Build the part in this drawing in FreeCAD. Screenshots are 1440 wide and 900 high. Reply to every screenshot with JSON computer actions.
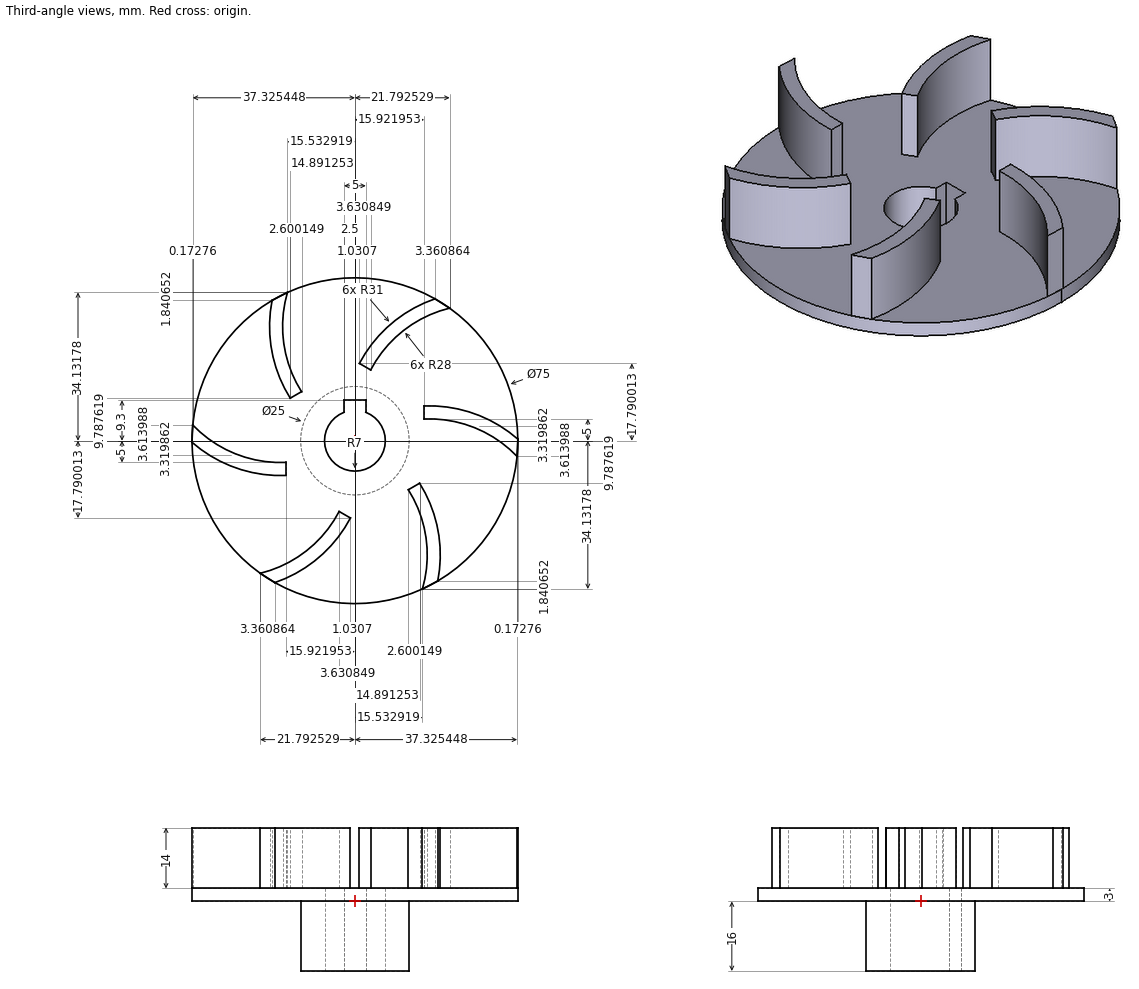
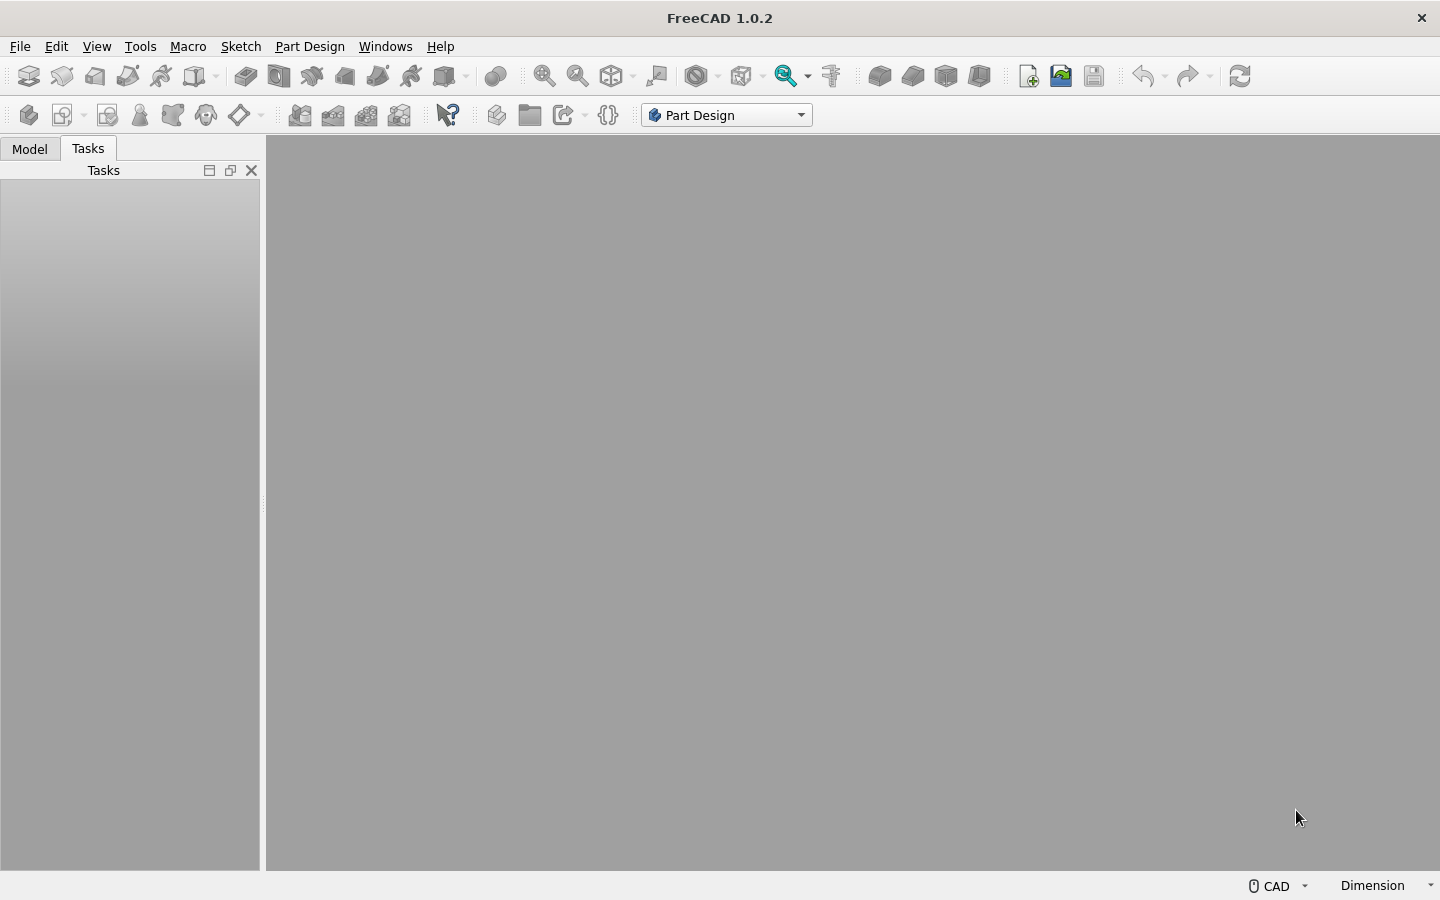
{"action": "key", "text": "ctrl+n"}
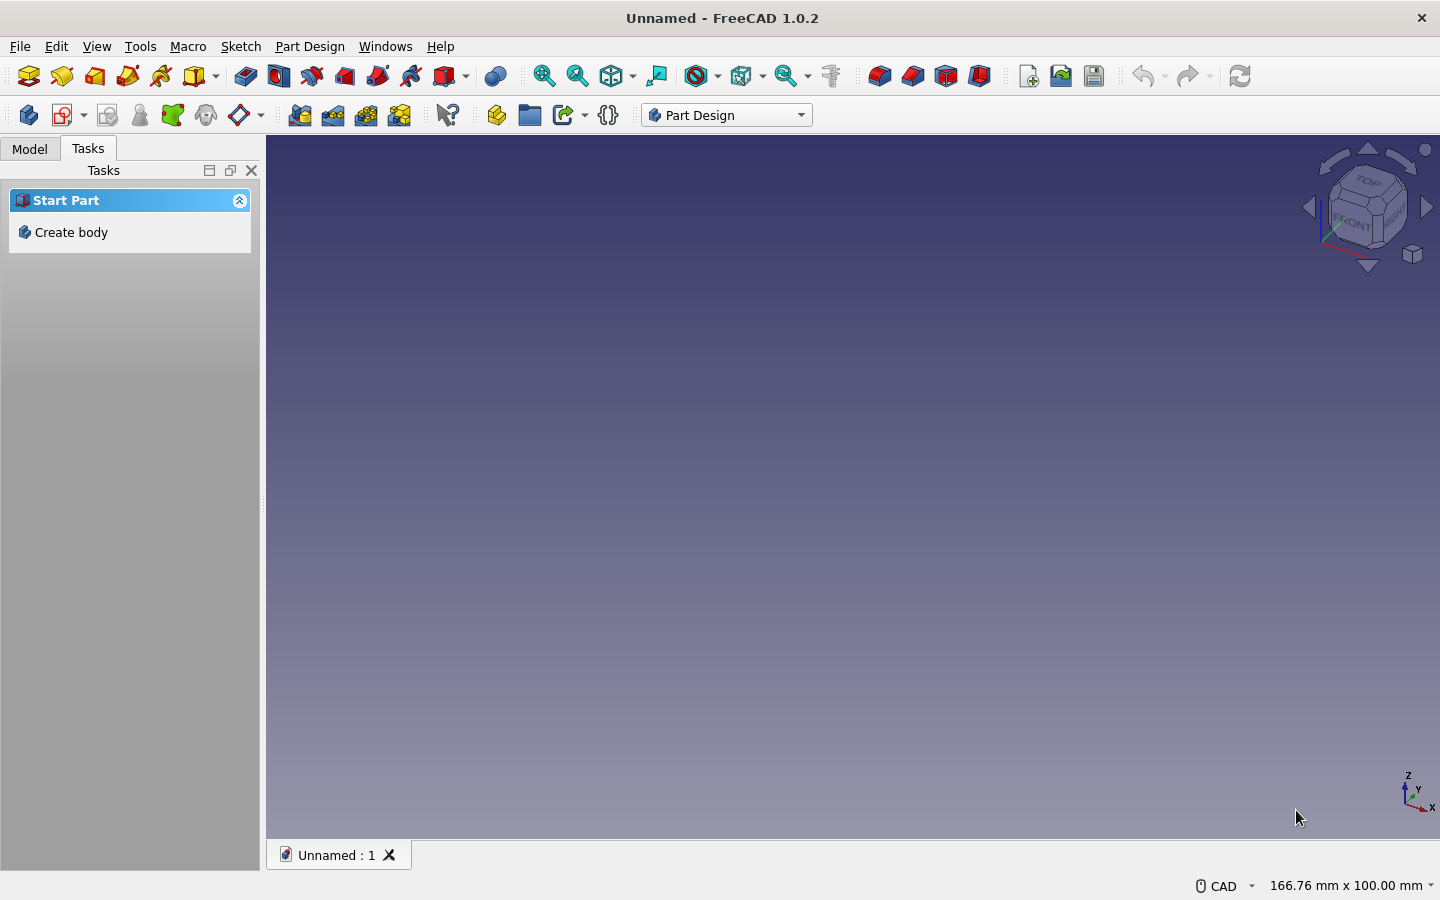
{"action": "left_click", "coordinate": [62, 116]}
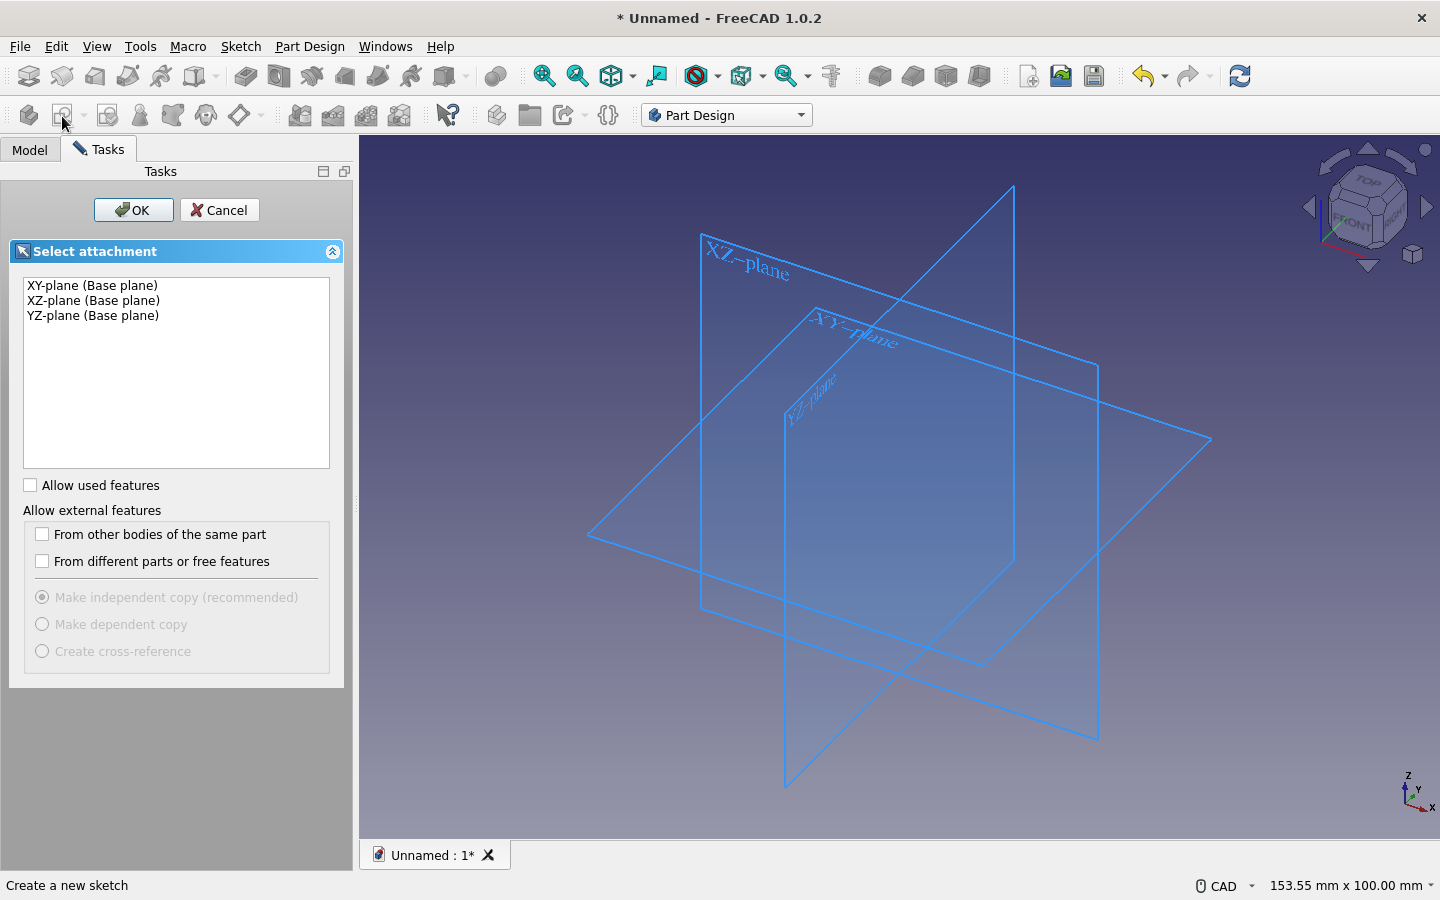
{"action": "left_click", "coordinate": [84, 286]}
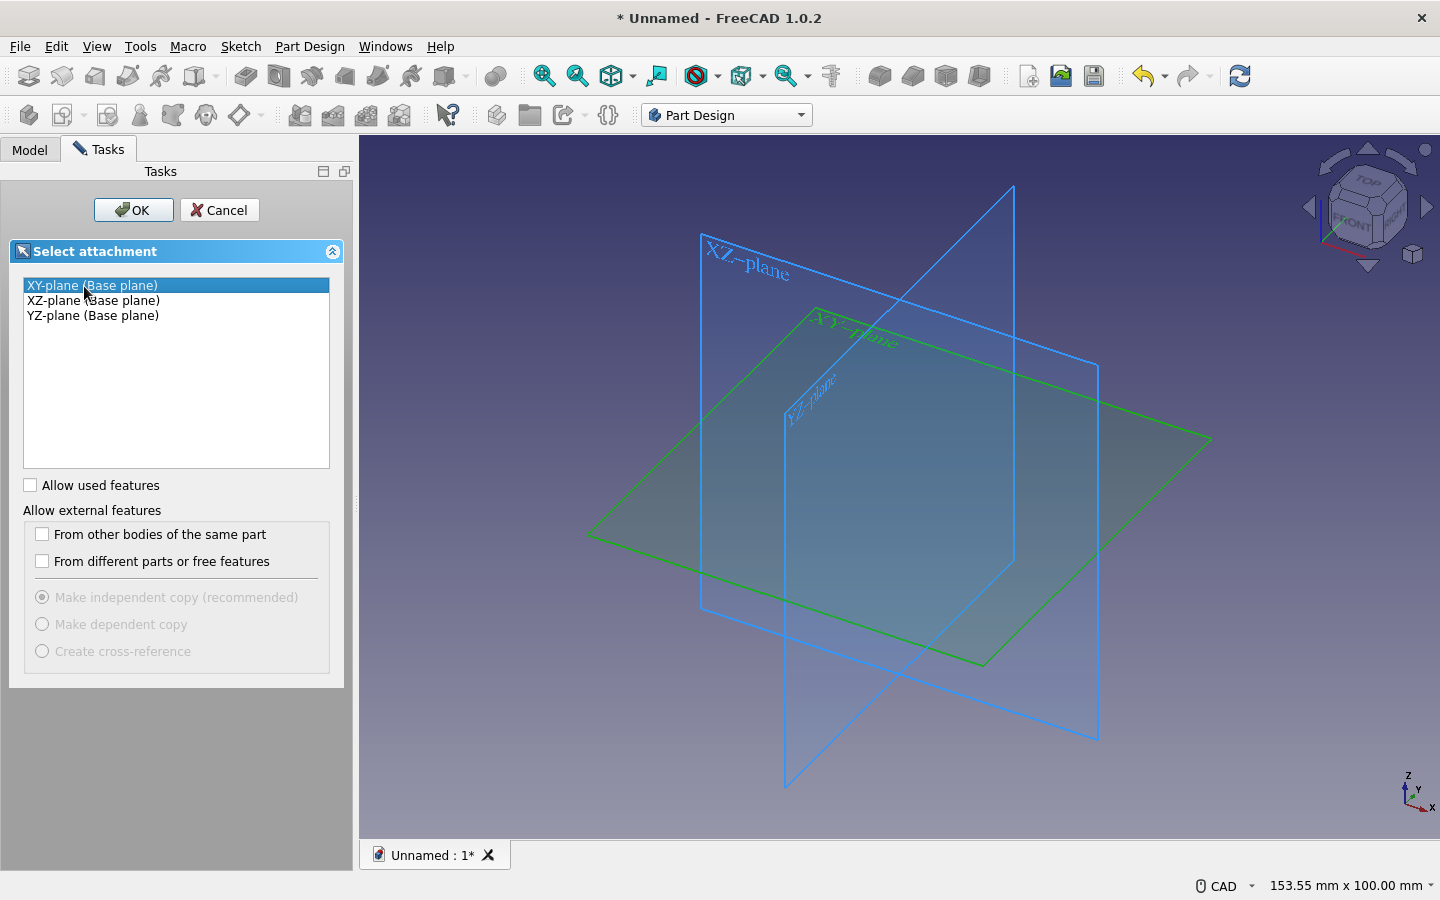
{"action": "left_click", "coordinate": [134, 210]}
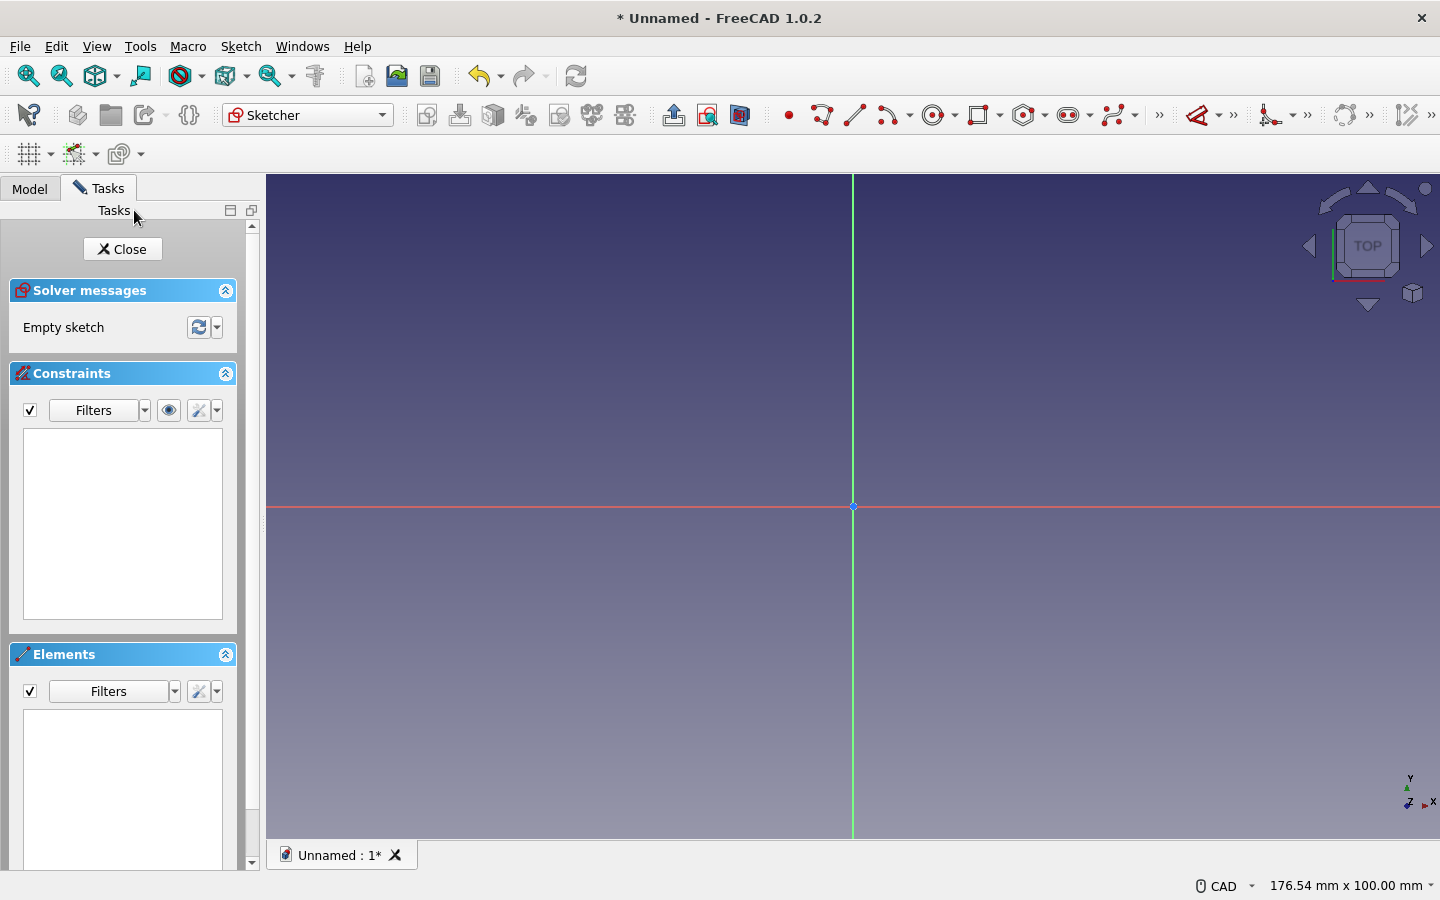
{"action": "key", "text": "g c"}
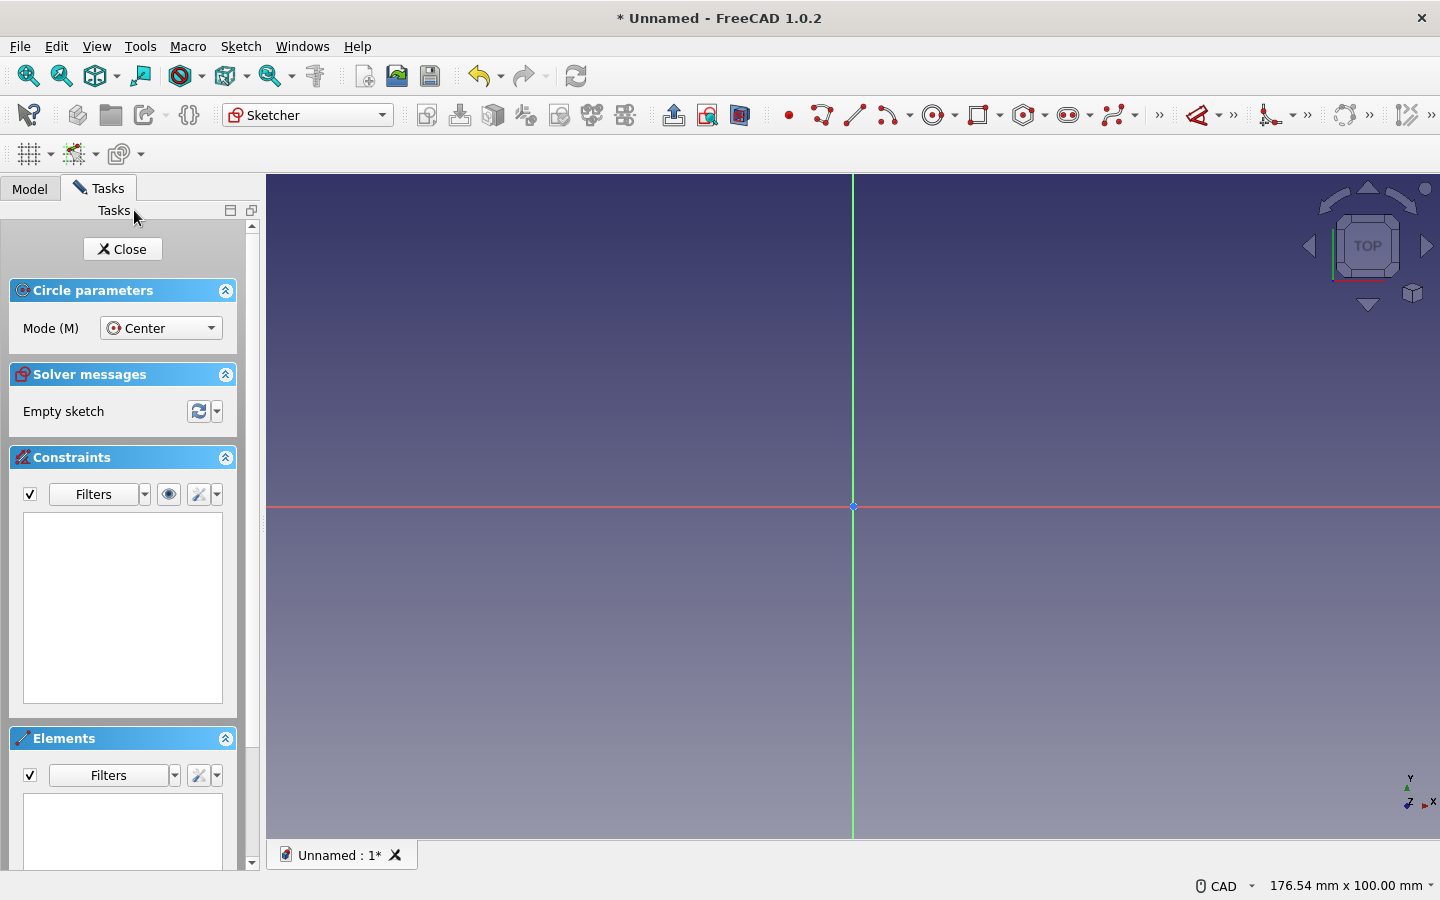
{"action": "left_click", "coordinate": [853, 506]}
{"action": "mouse_move", "coordinate": [1029, 330]}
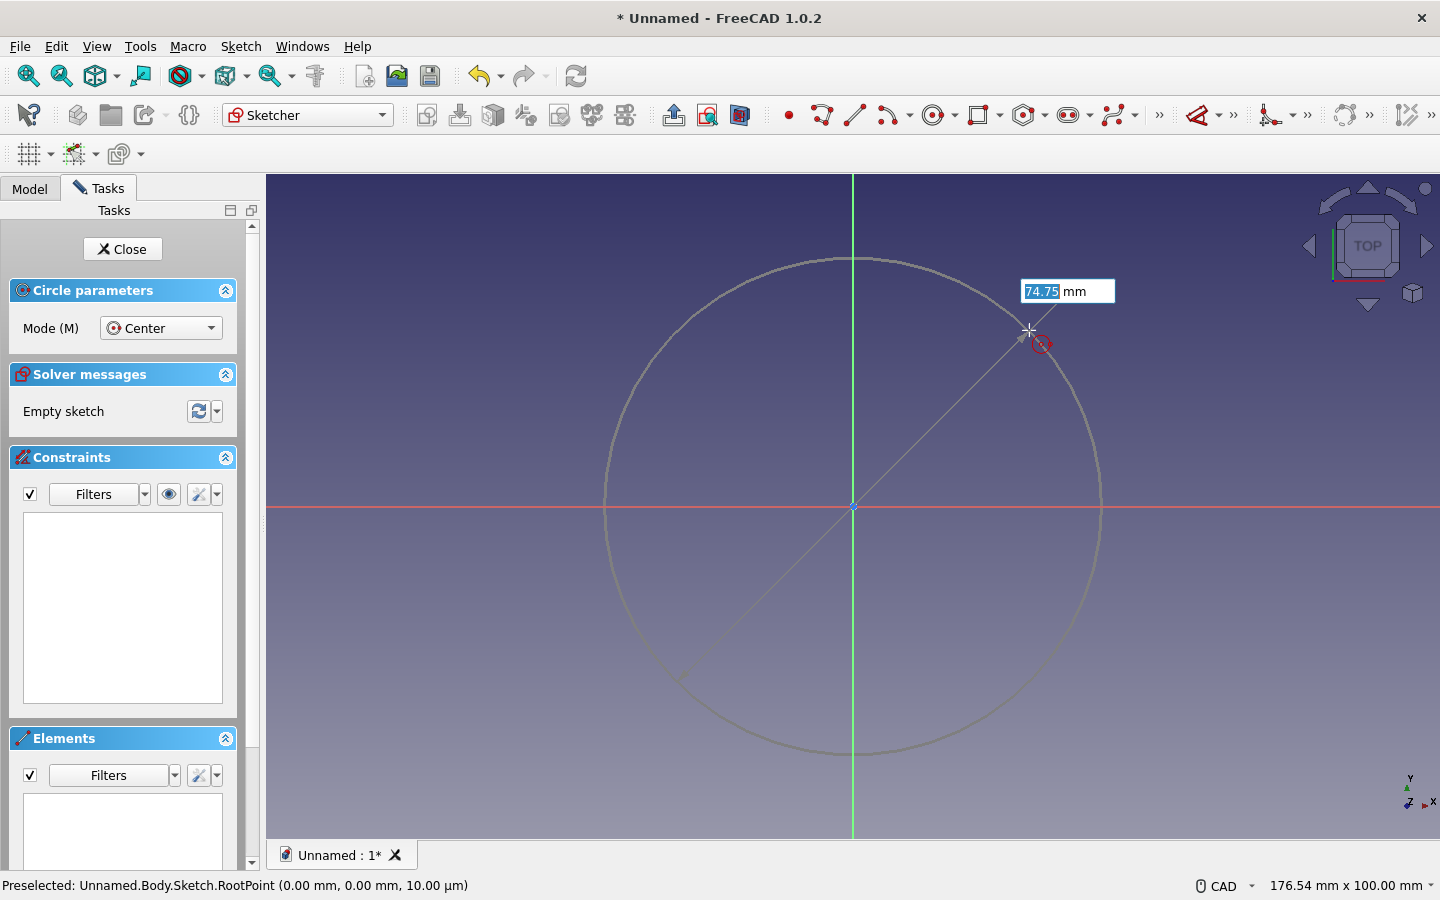
{"action": "type", "text": "75"}
{"action": "key", "text": "Return"}
{"action": "key", "text": "Escape"}